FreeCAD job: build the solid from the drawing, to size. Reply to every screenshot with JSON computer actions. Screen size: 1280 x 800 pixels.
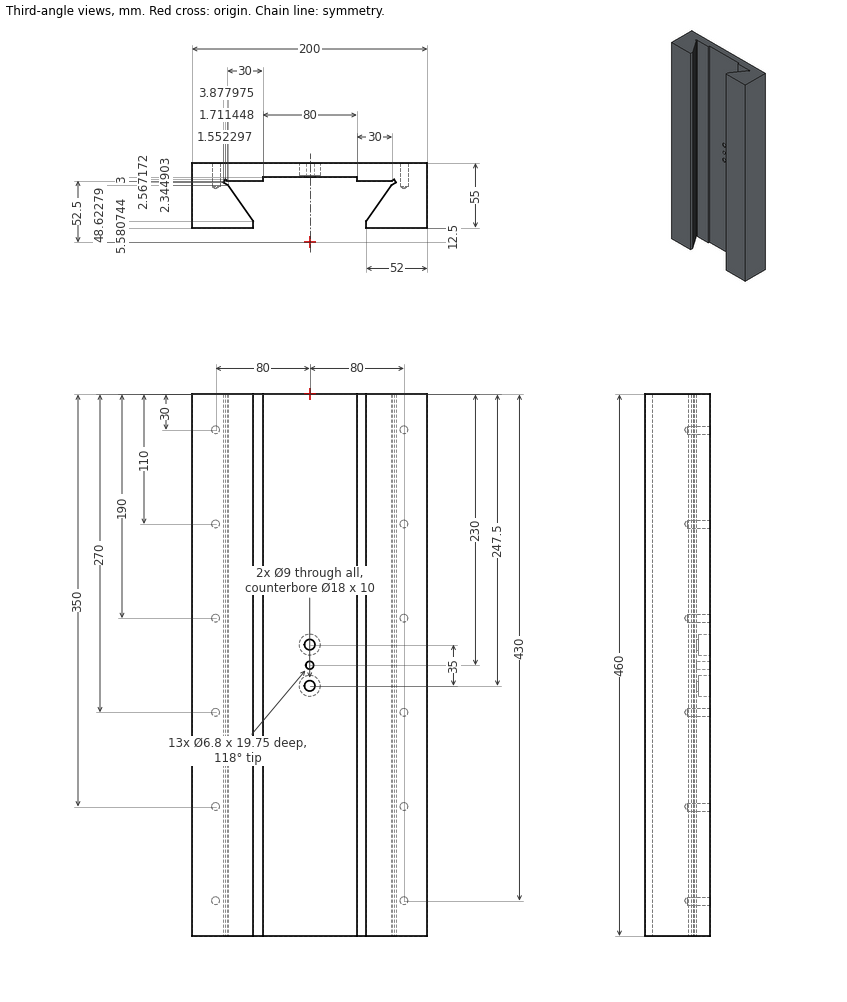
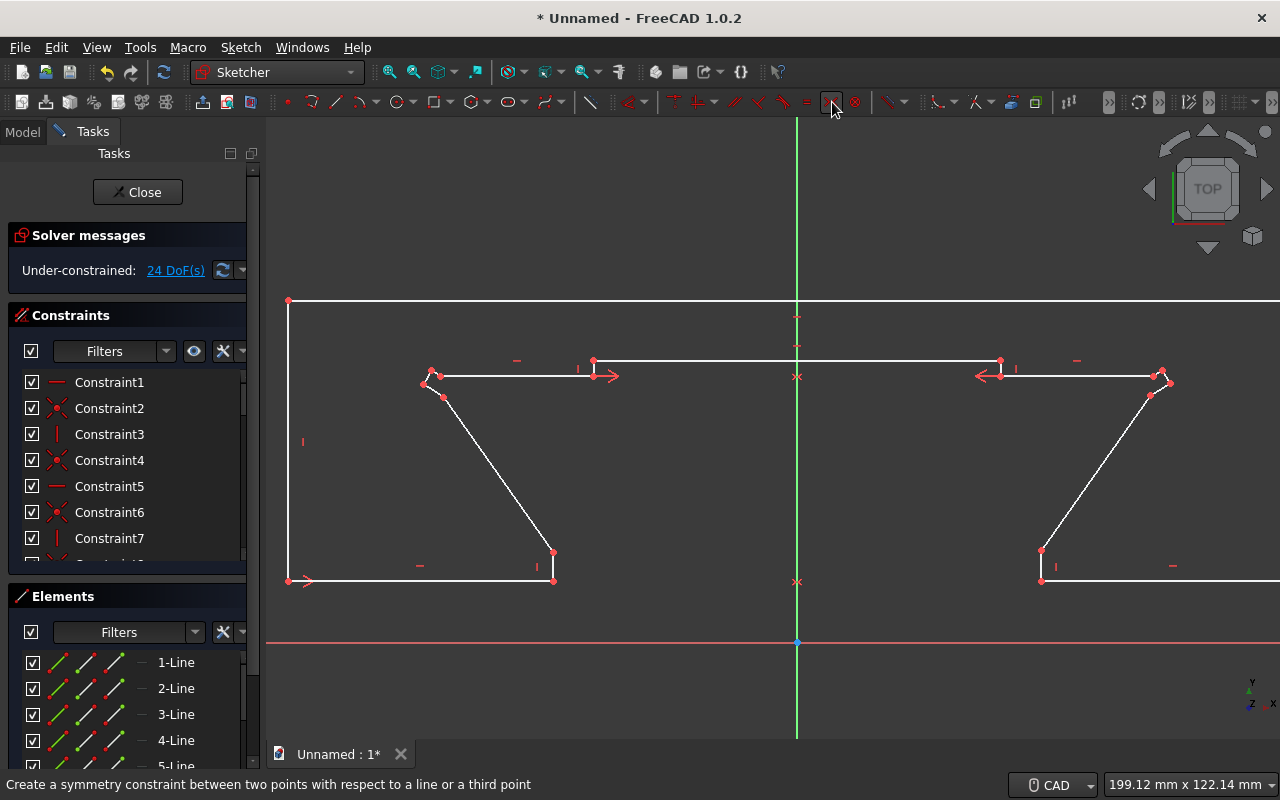
{"action": "left_click", "coordinate": [432, 371]}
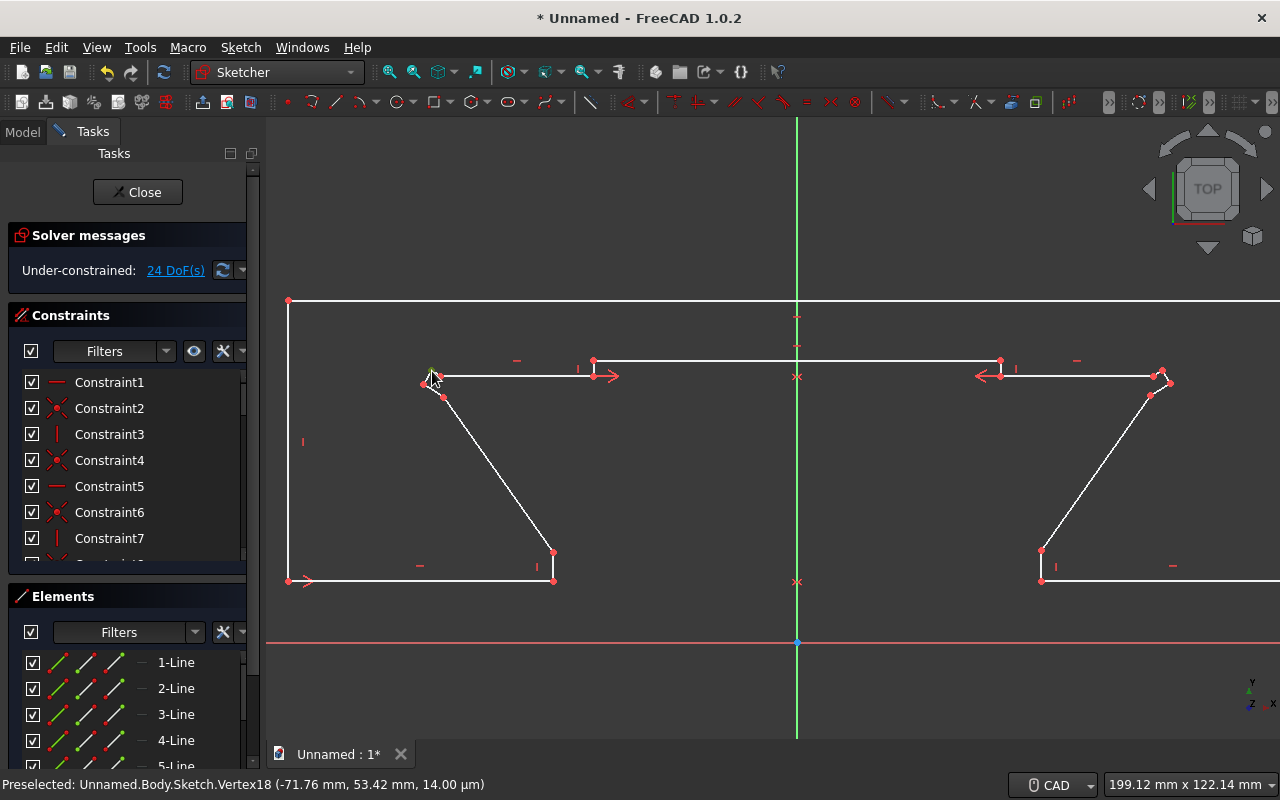
{"action": "scroll", "coordinate": [592, 376], "scroll_direction": "down", "scroll_amount": 3}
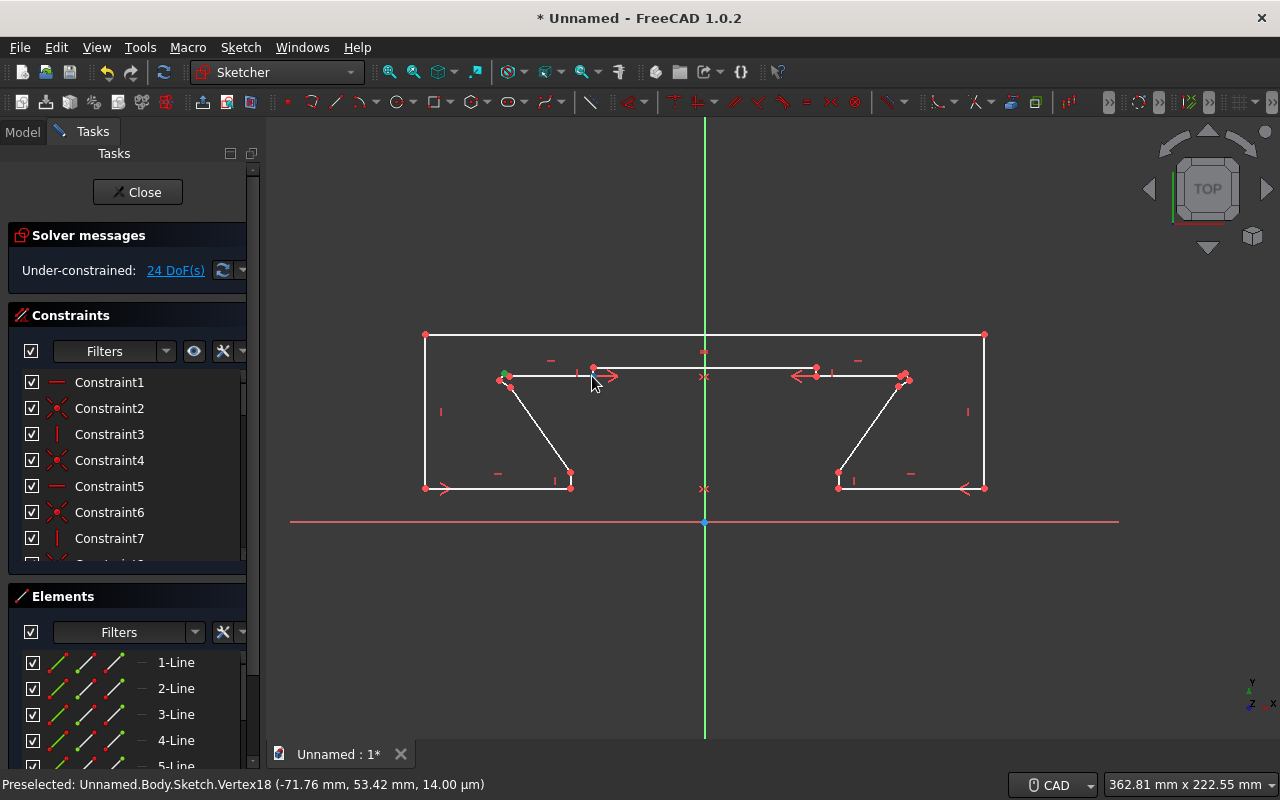
{"action": "scroll", "coordinate": [905, 373], "scroll_direction": "up", "scroll_amount": 4}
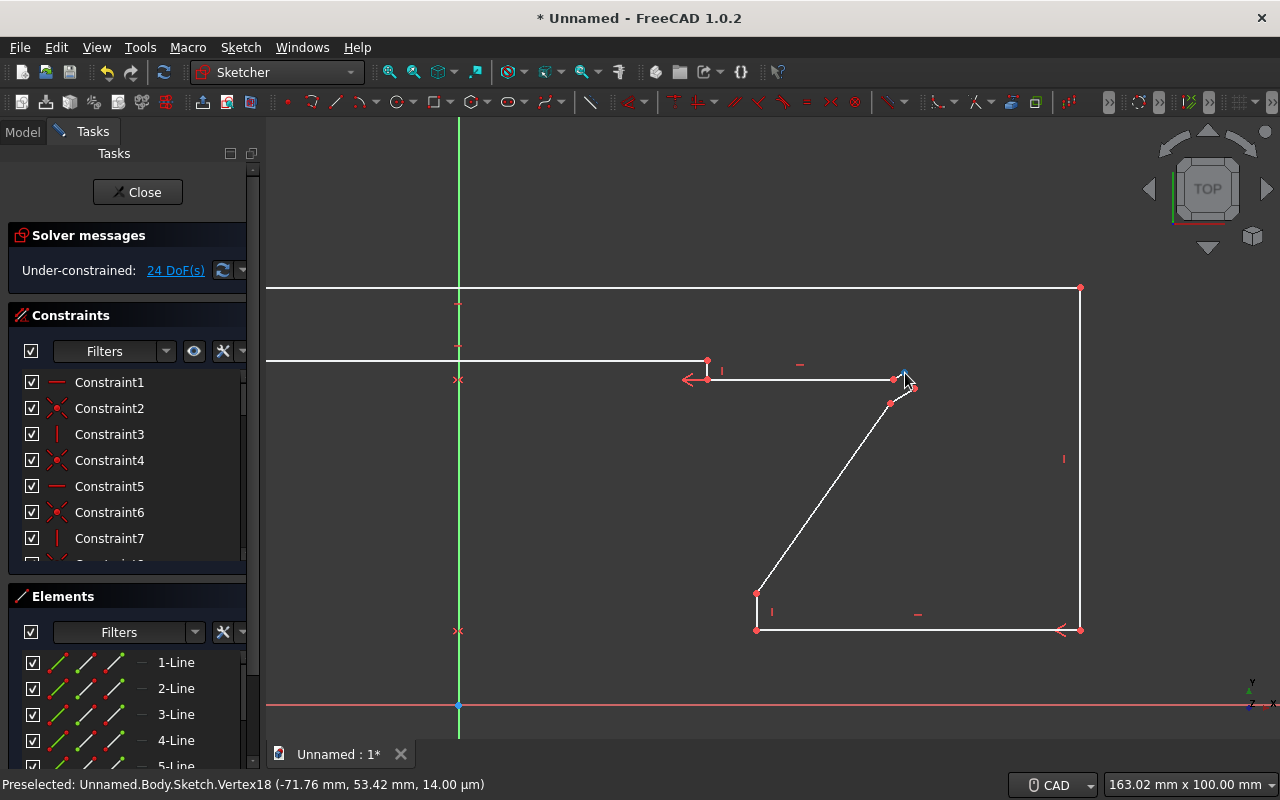
{"action": "left_click", "coordinate": [904, 373]}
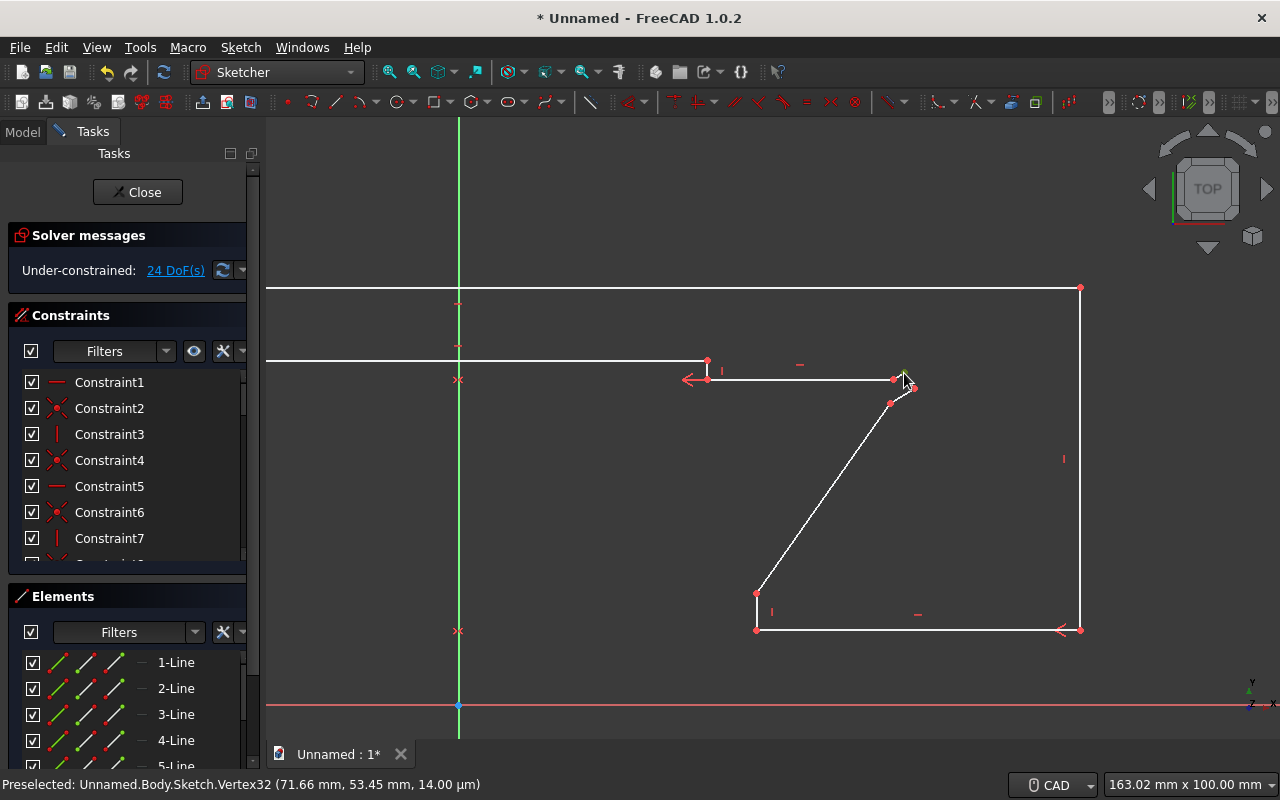
{"action": "left_click", "coordinate": [459, 671]}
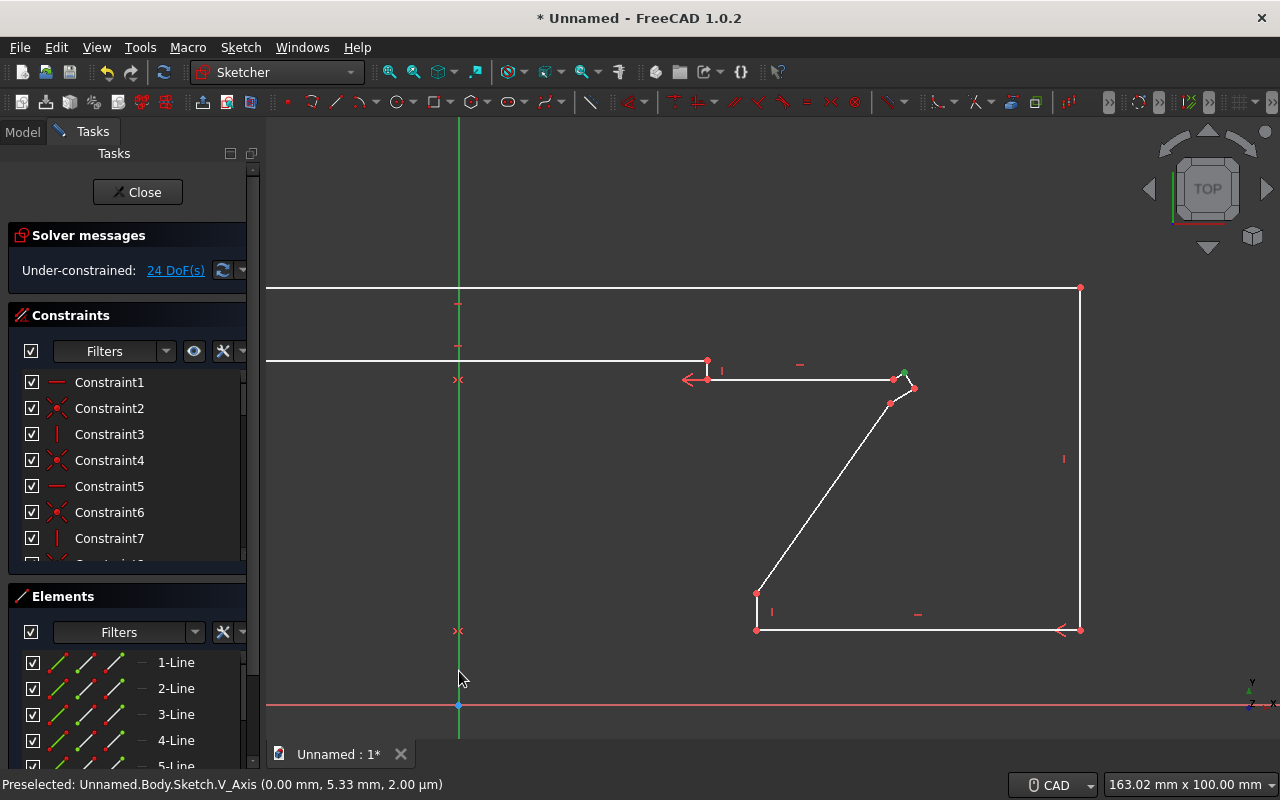
{"action": "left_click", "coordinate": [832, 102]}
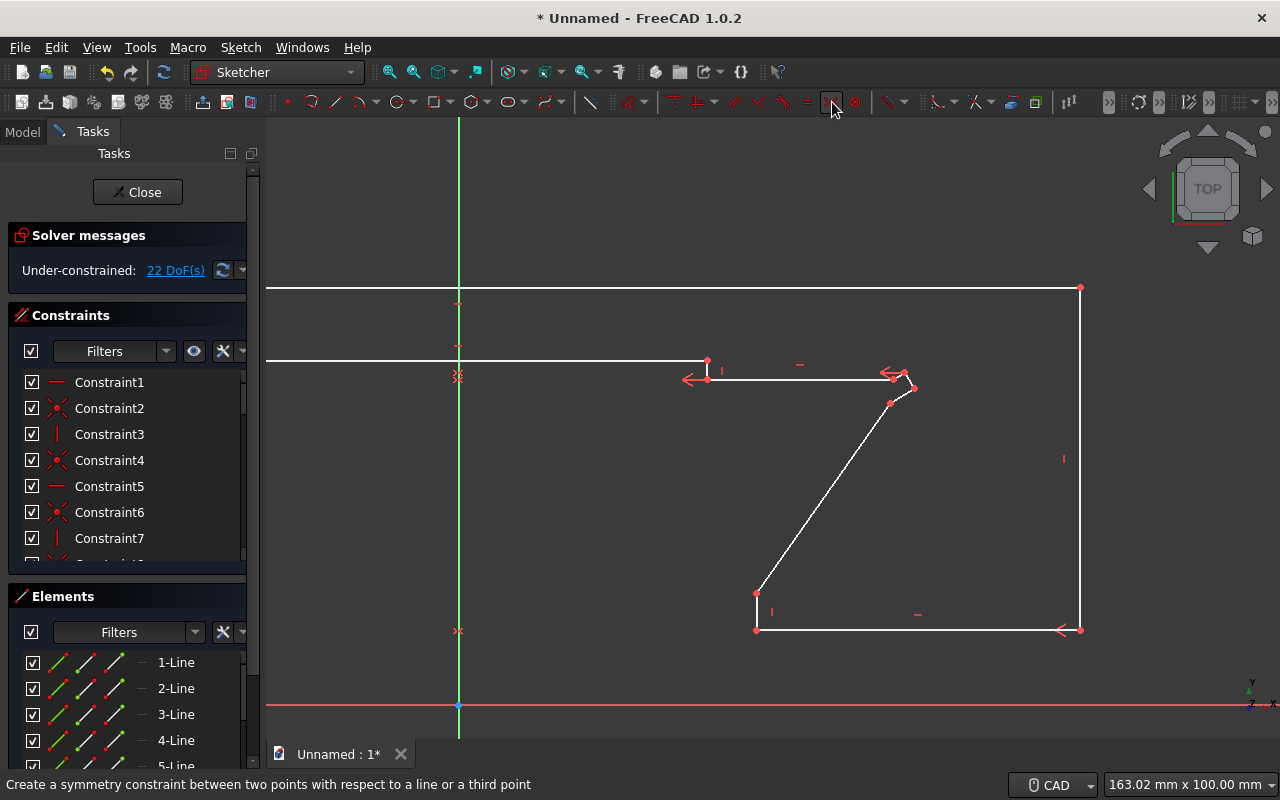
{"action": "scroll", "coordinate": [905, 373], "scroll_direction": "down", "scroll_amount": 4}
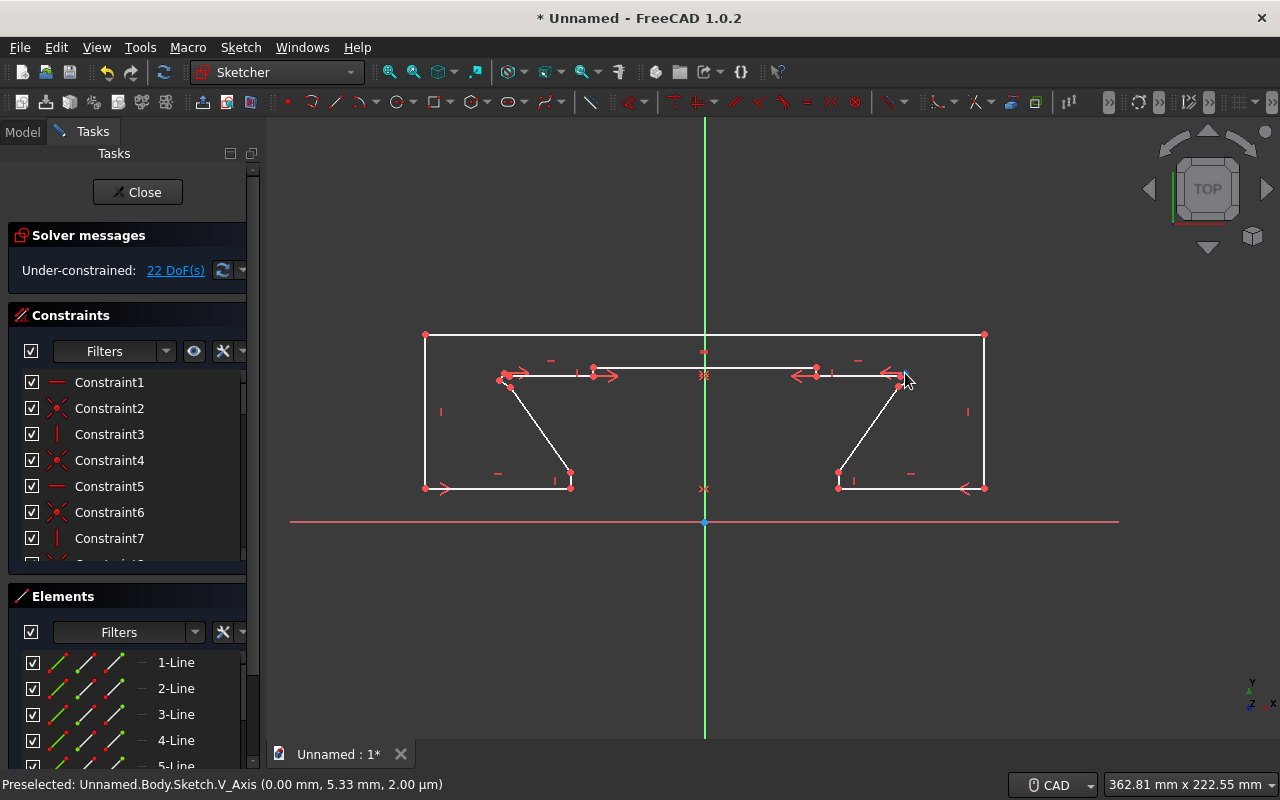
{"action": "scroll", "coordinate": [500, 381], "scroll_direction": "up", "scroll_amount": 2}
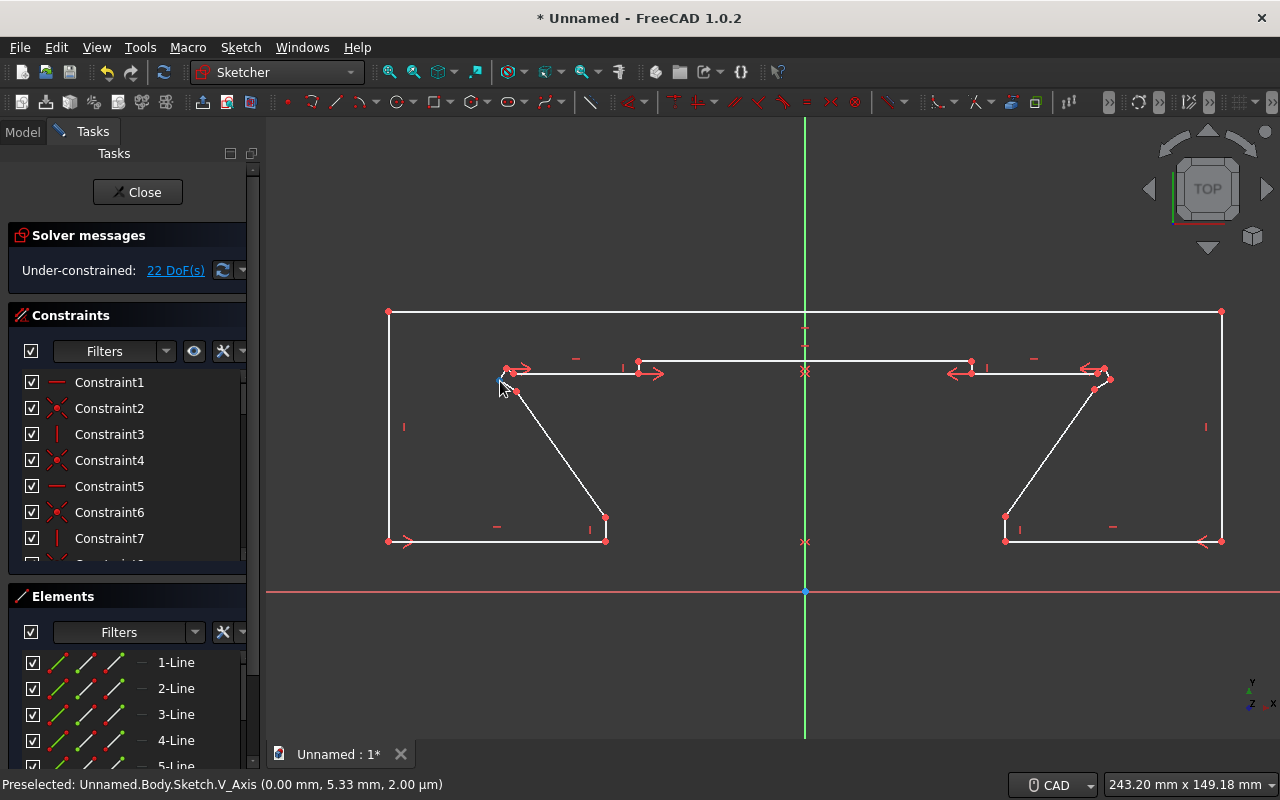
{"action": "left_click", "coordinate": [500, 380]}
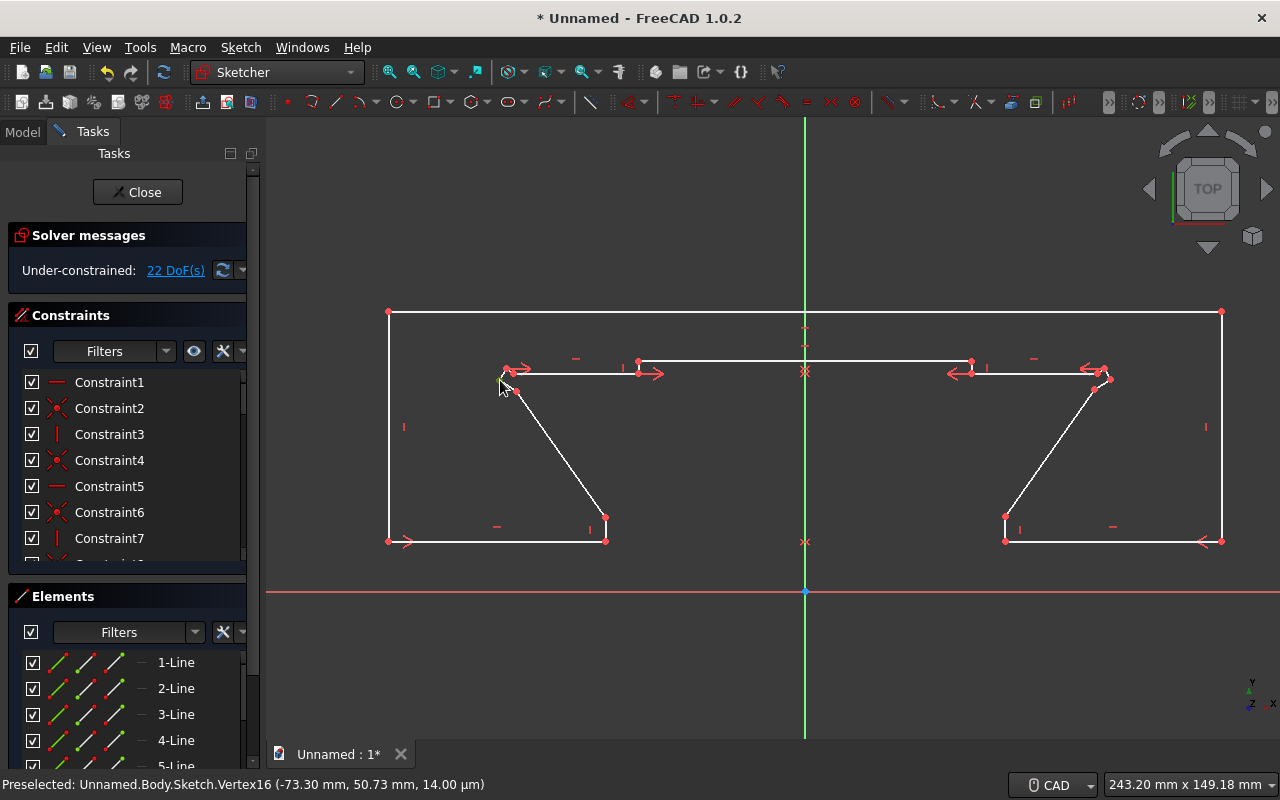
{"action": "left_click", "coordinate": [1111, 380]}